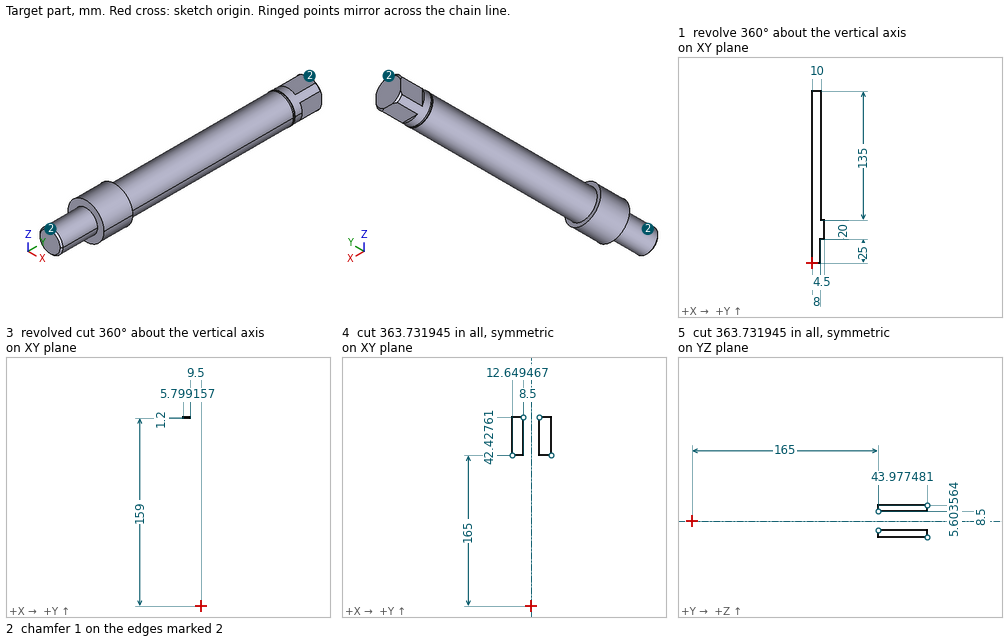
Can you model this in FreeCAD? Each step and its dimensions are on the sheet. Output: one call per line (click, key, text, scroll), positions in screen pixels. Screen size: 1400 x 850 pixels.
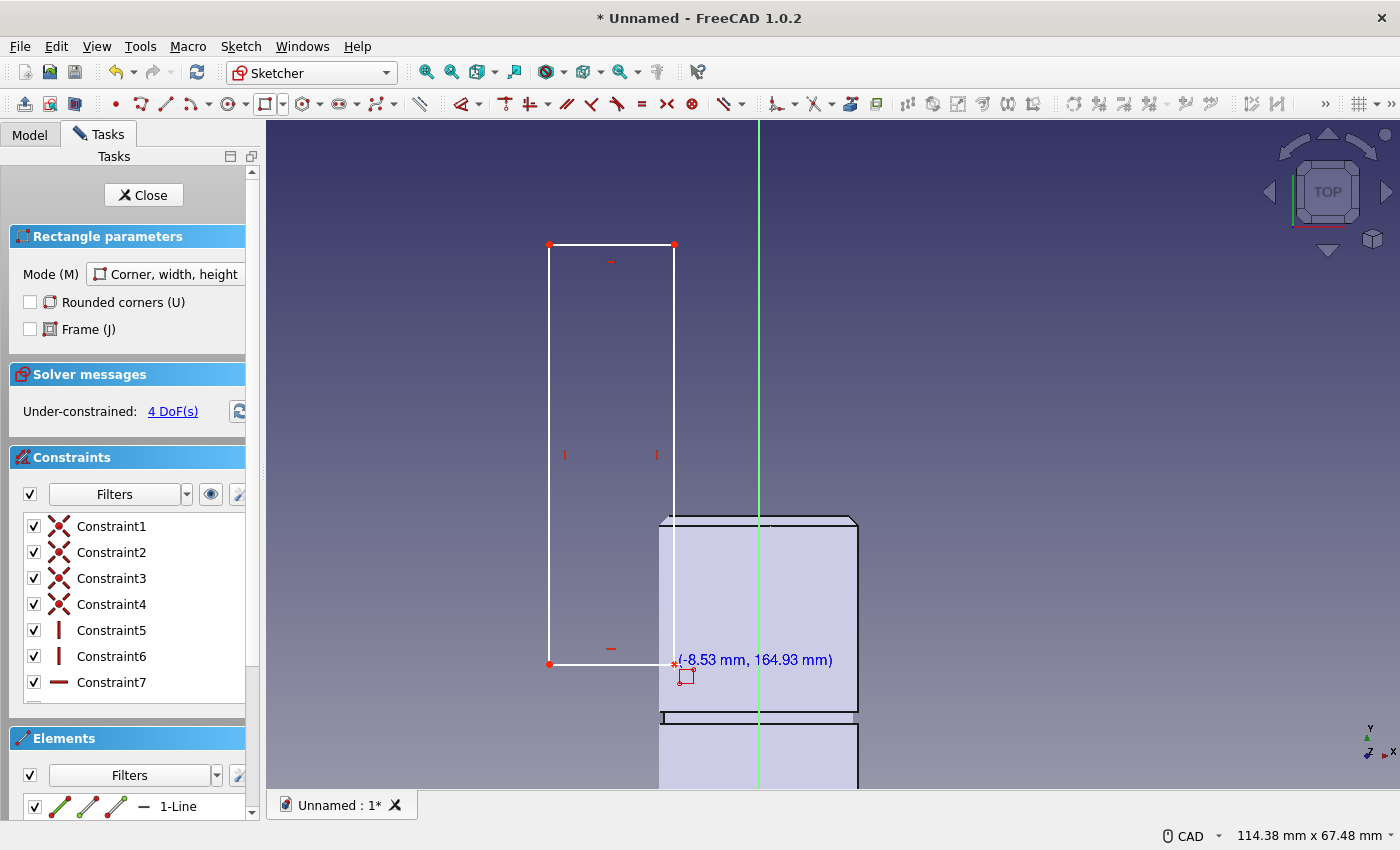
click(843, 244)
click(968, 664)
key(Escape)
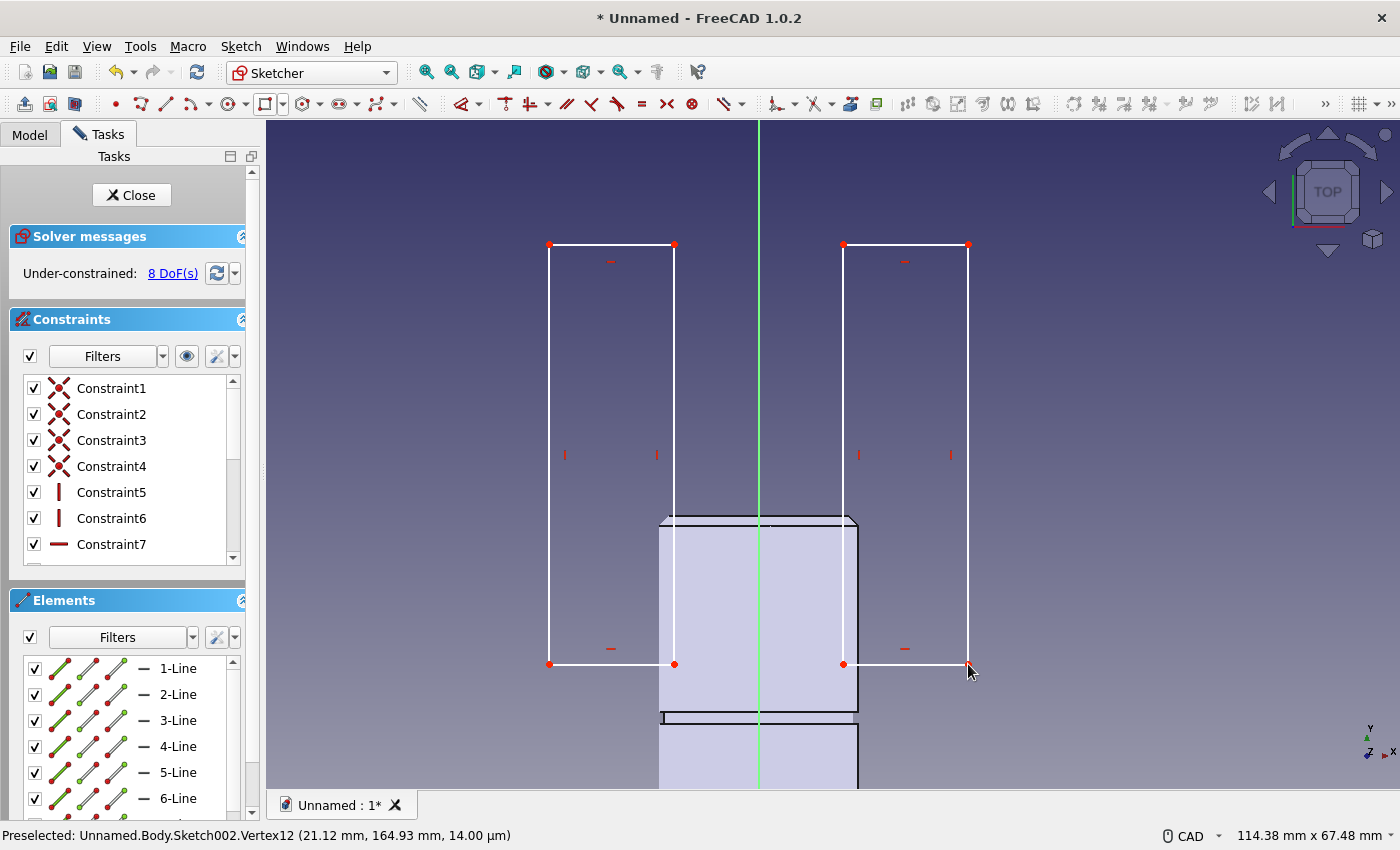
click(674, 245)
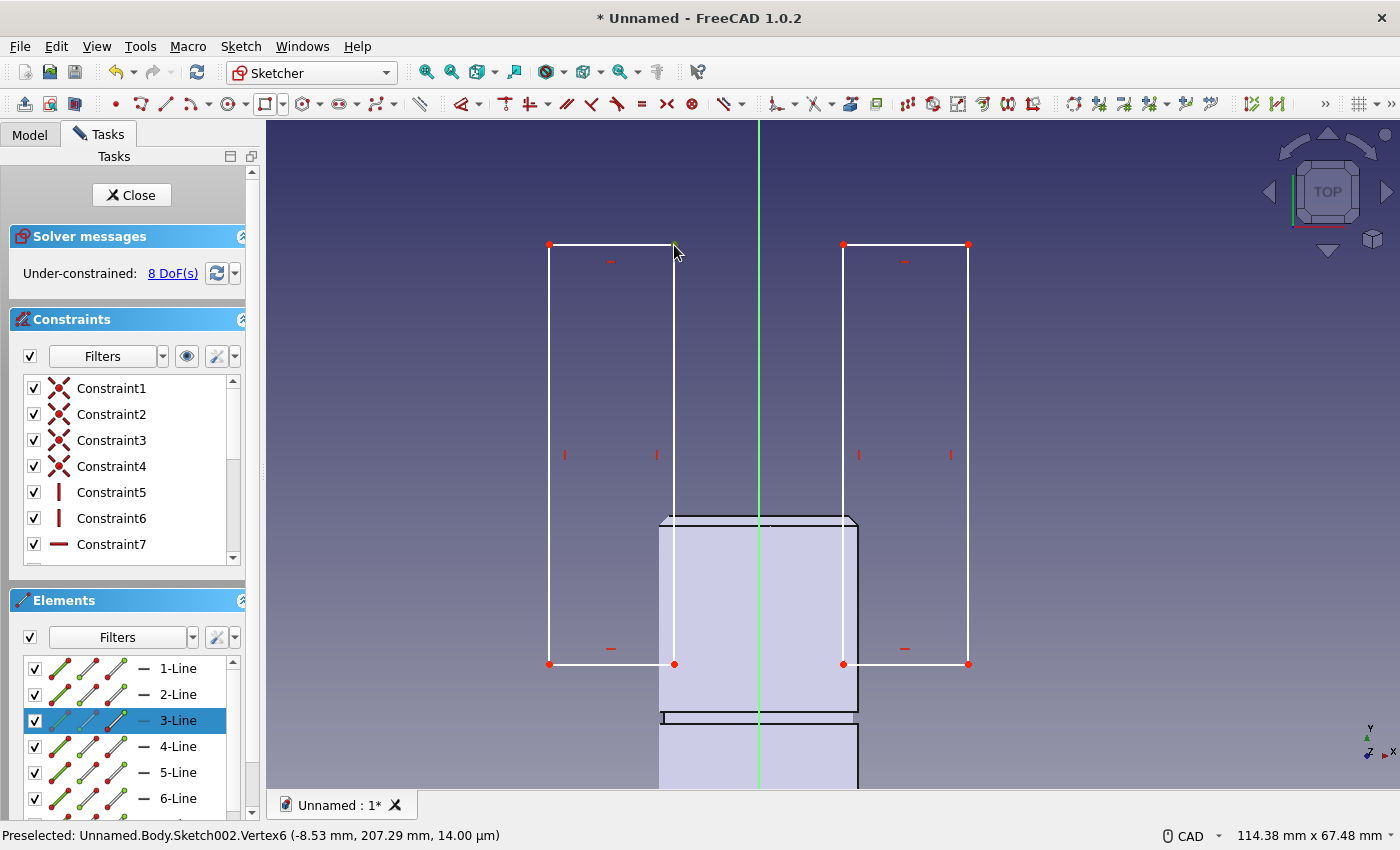
click(843, 245)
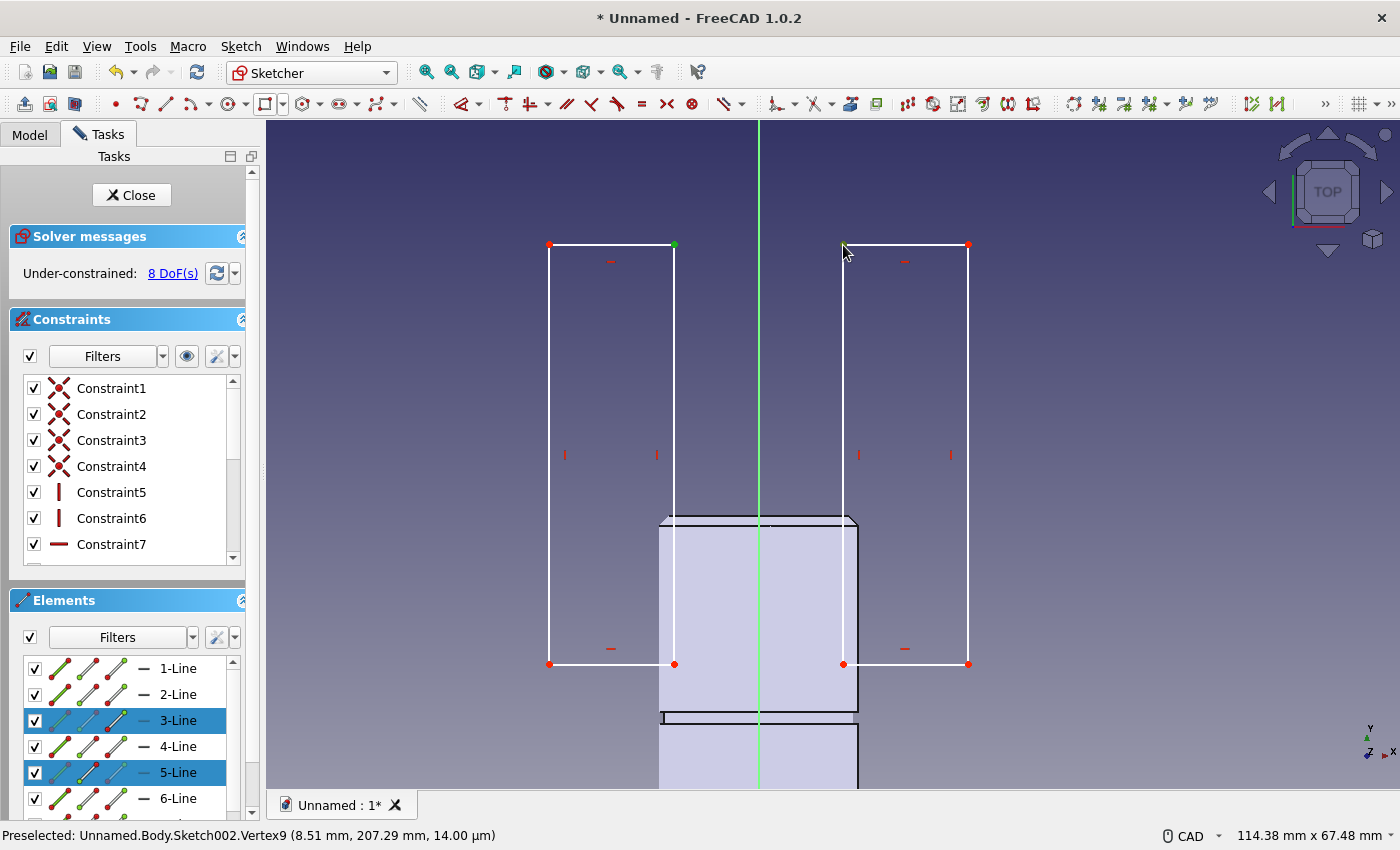
click(759, 717)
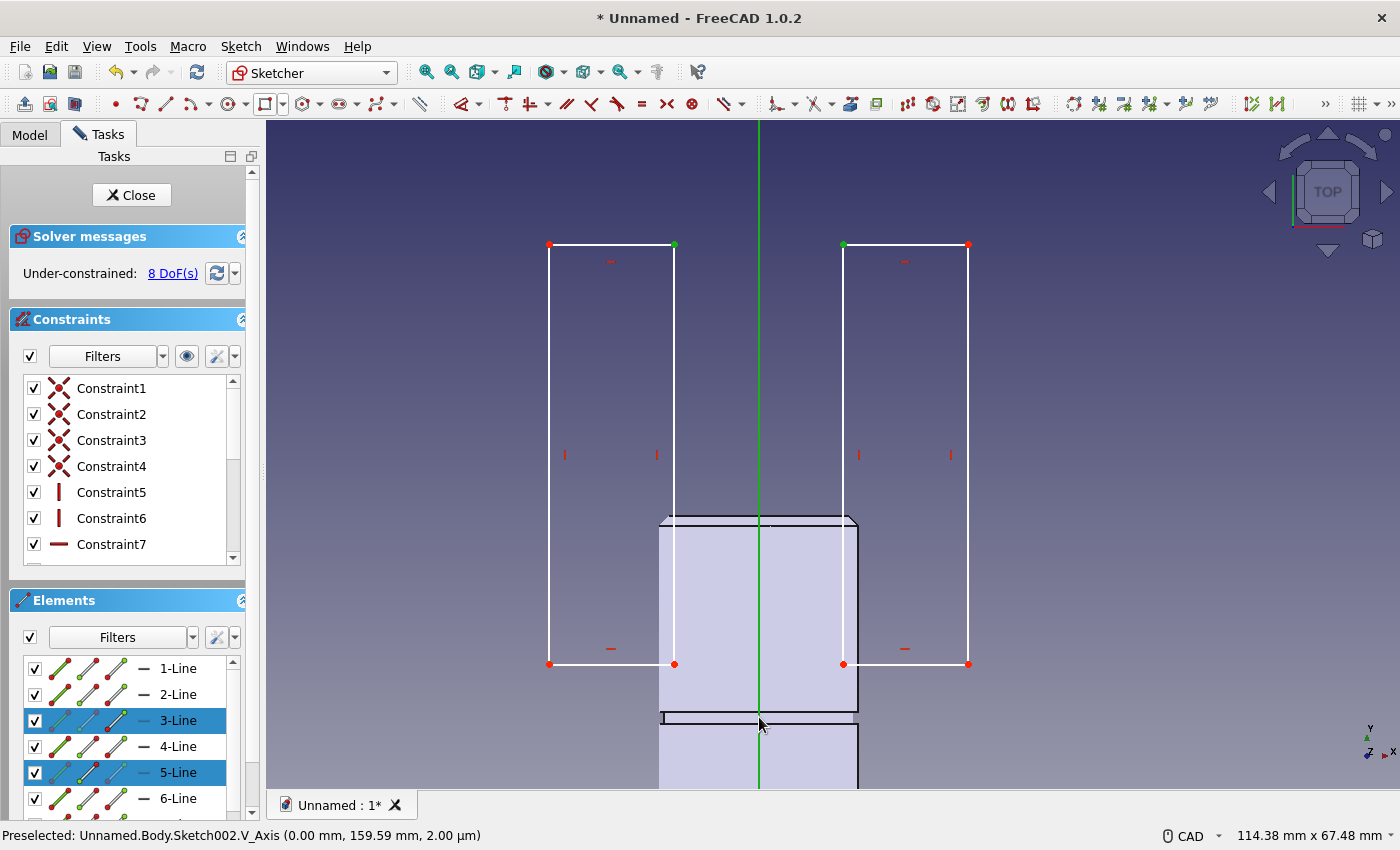
click(667, 104)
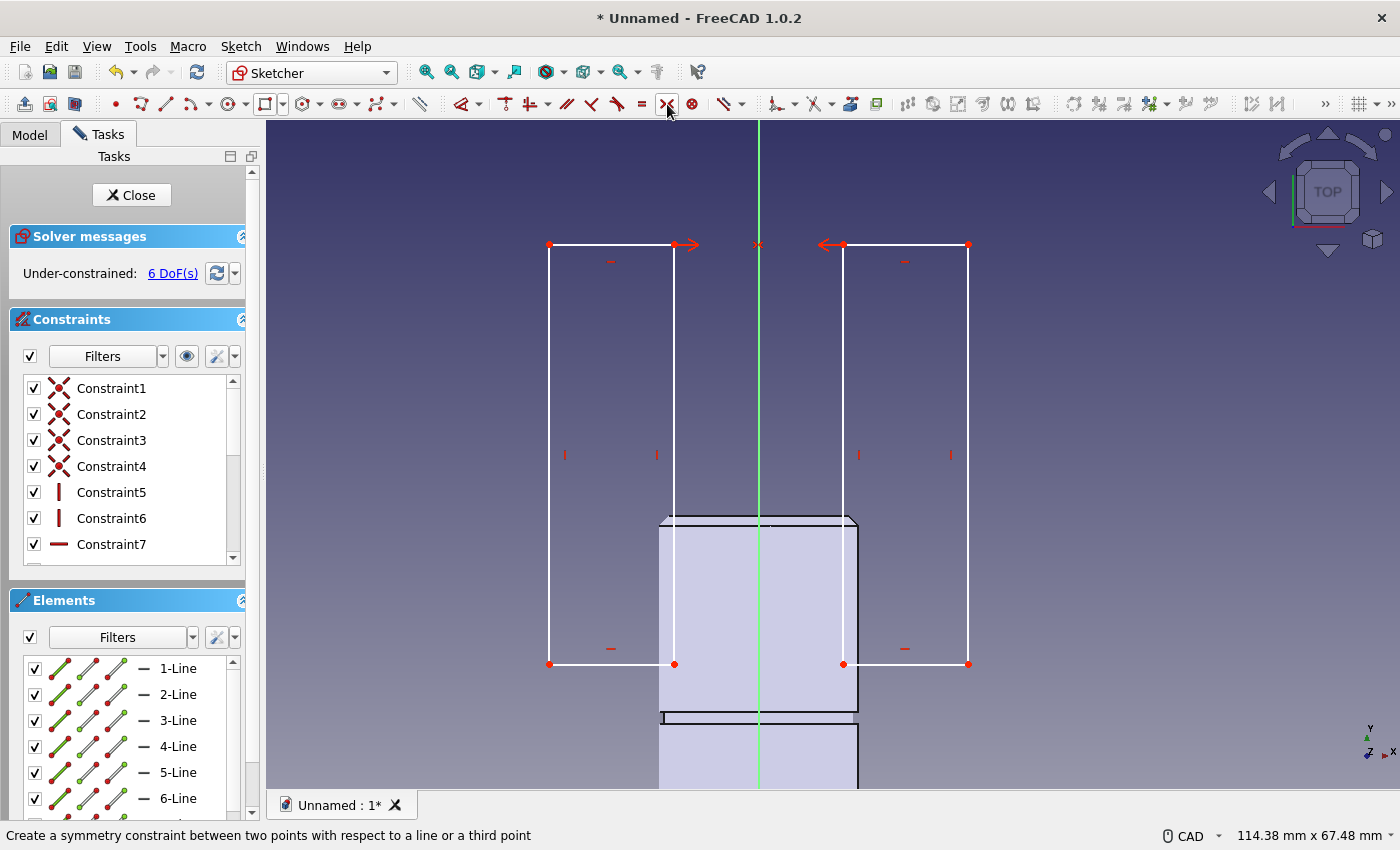
click(549, 665)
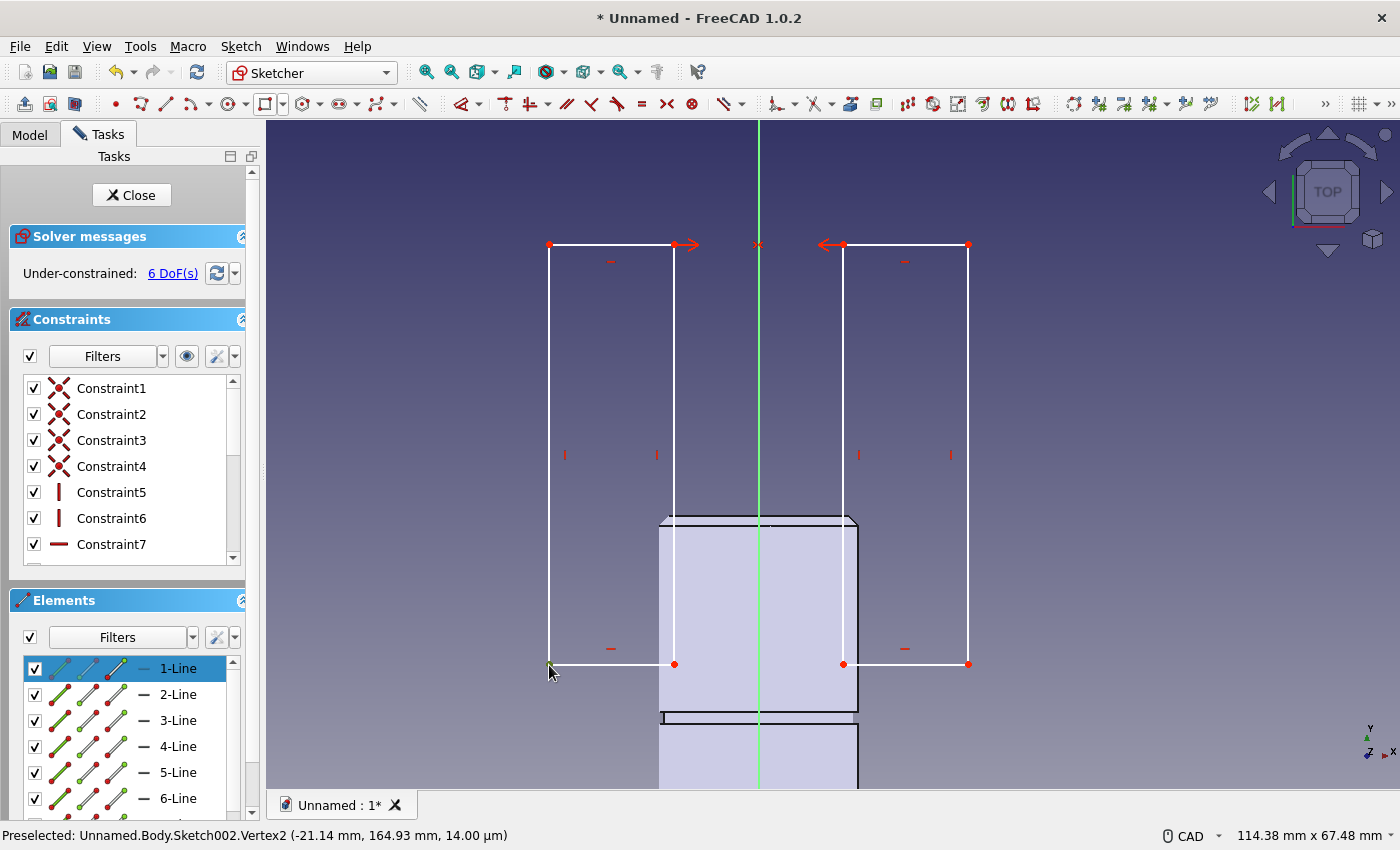
click(968, 665)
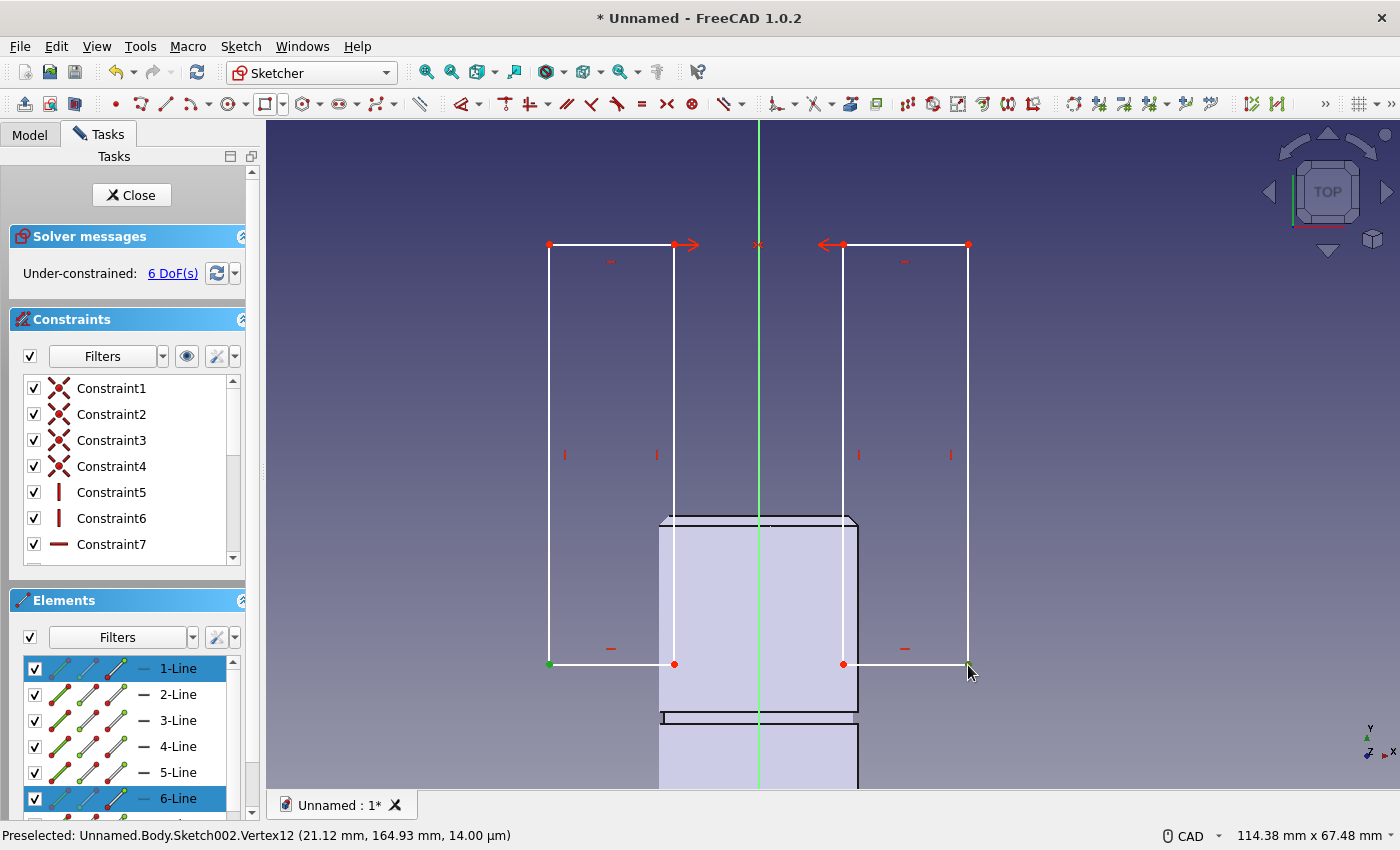
click(759, 717)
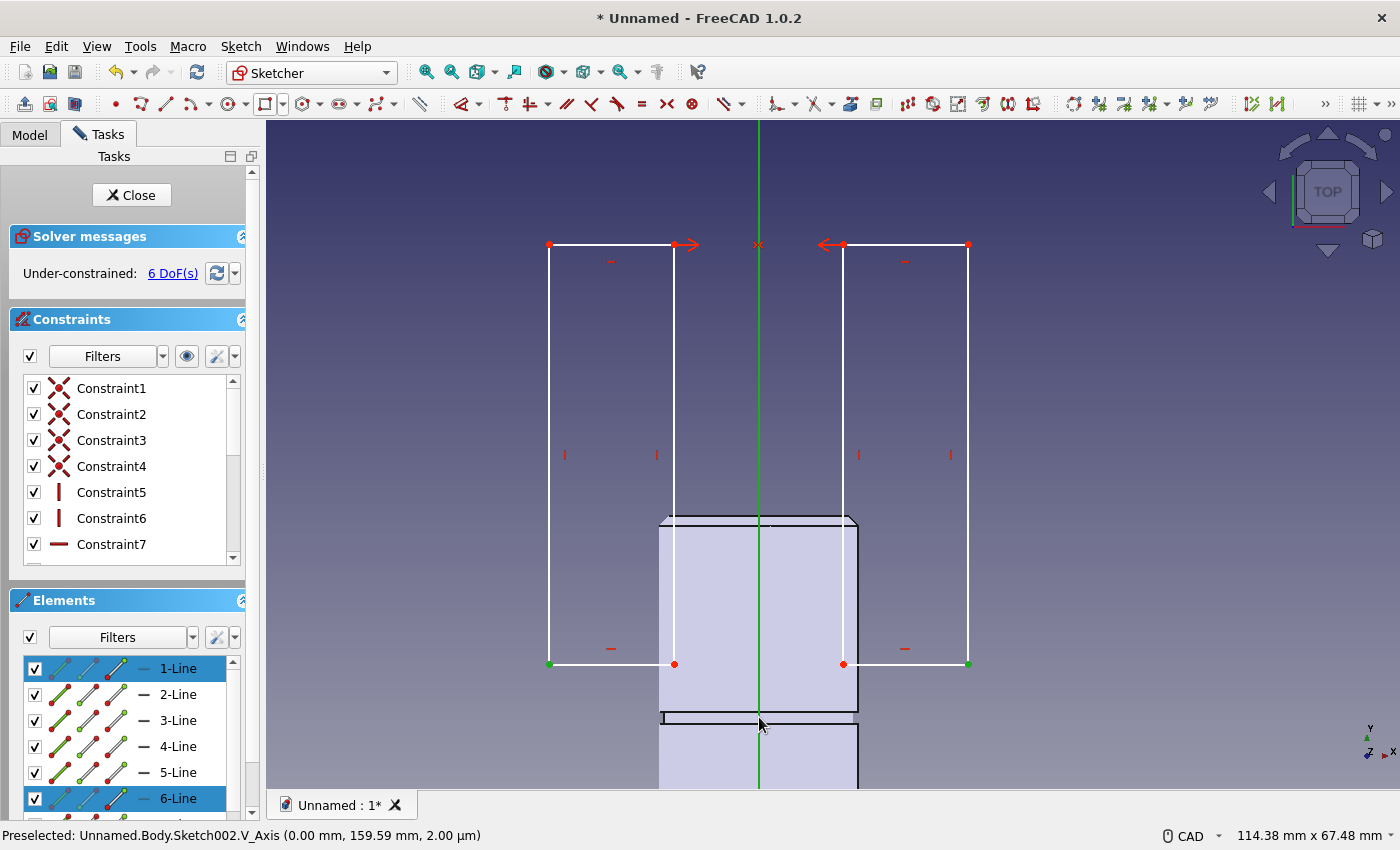
key(s)